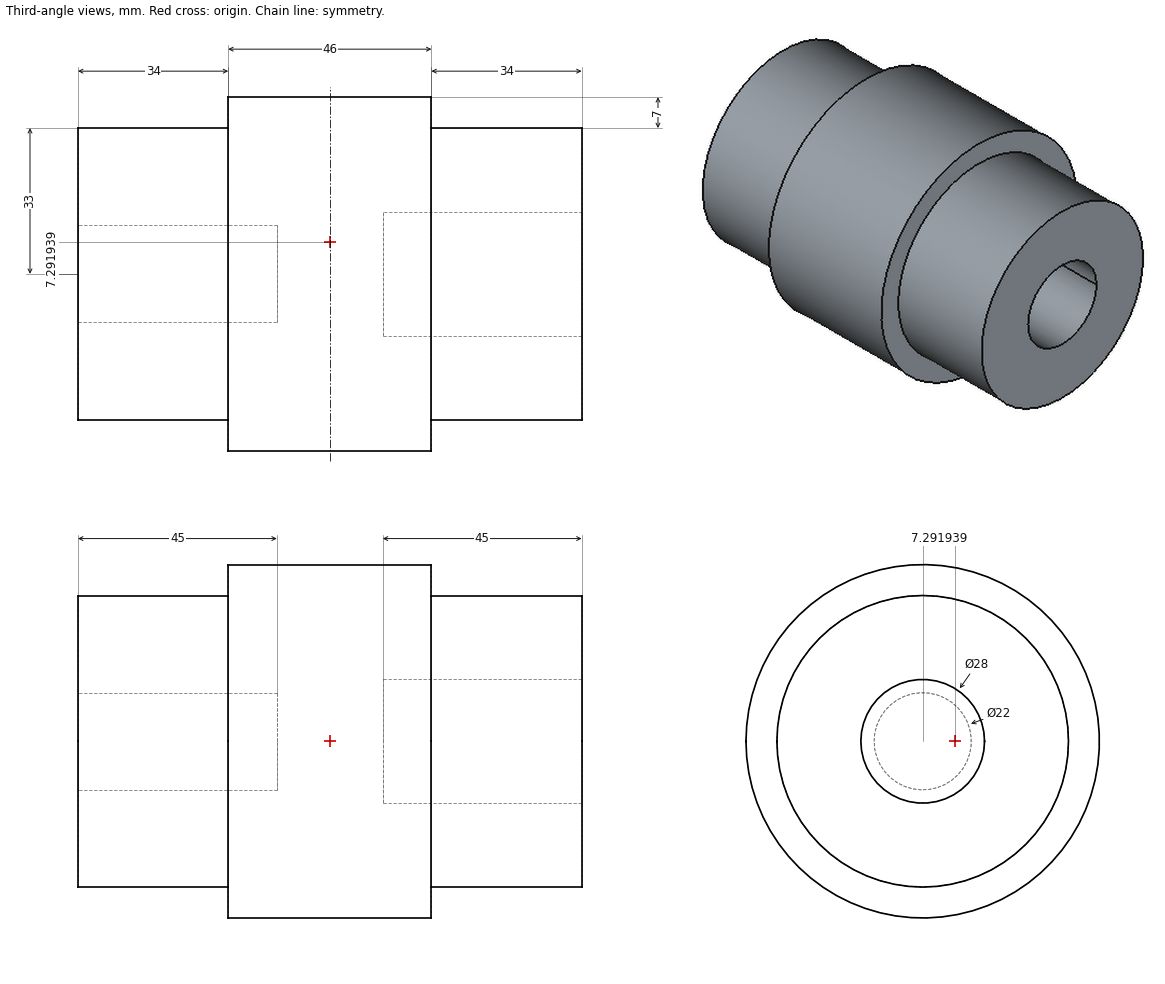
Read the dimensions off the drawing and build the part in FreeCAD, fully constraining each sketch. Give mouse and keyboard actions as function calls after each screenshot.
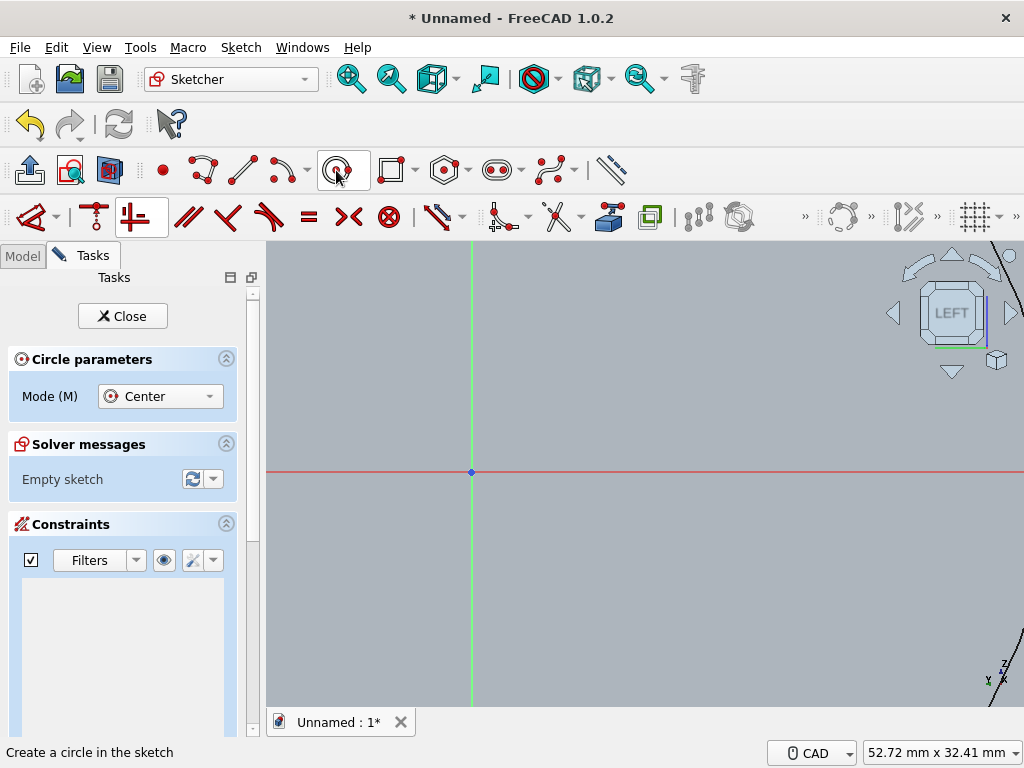
click(577, 472)
move(688, 360)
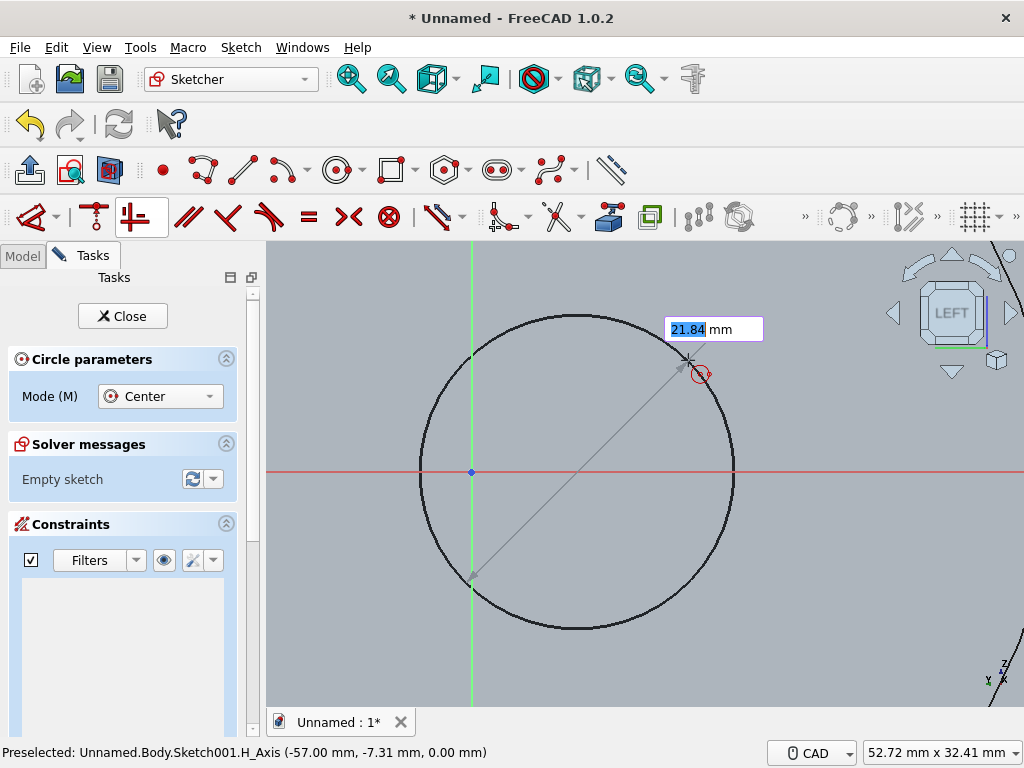
text(22)
key(Return)
key(Escape)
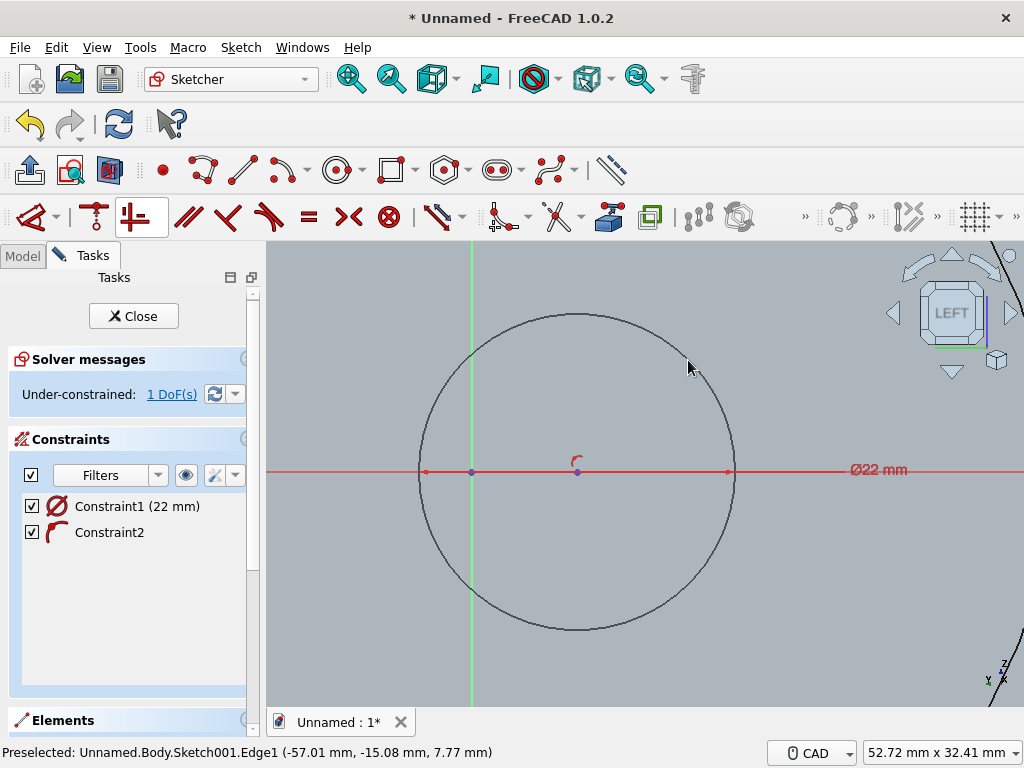
click(32, 218)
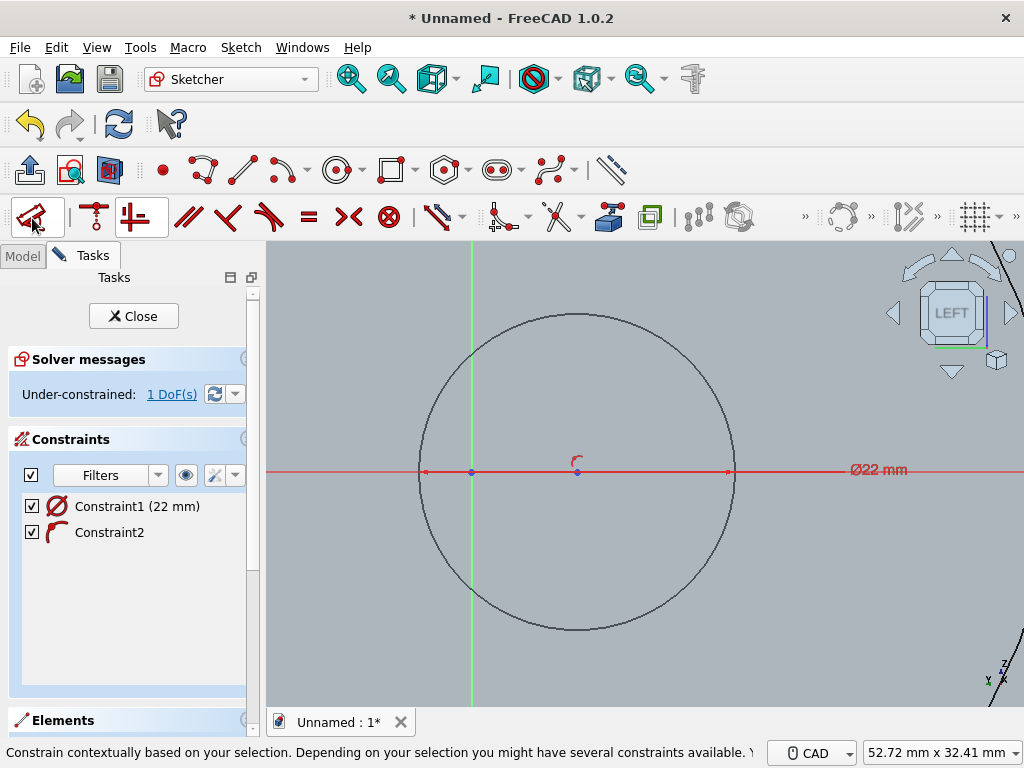
click(577, 472)
click(524, 506)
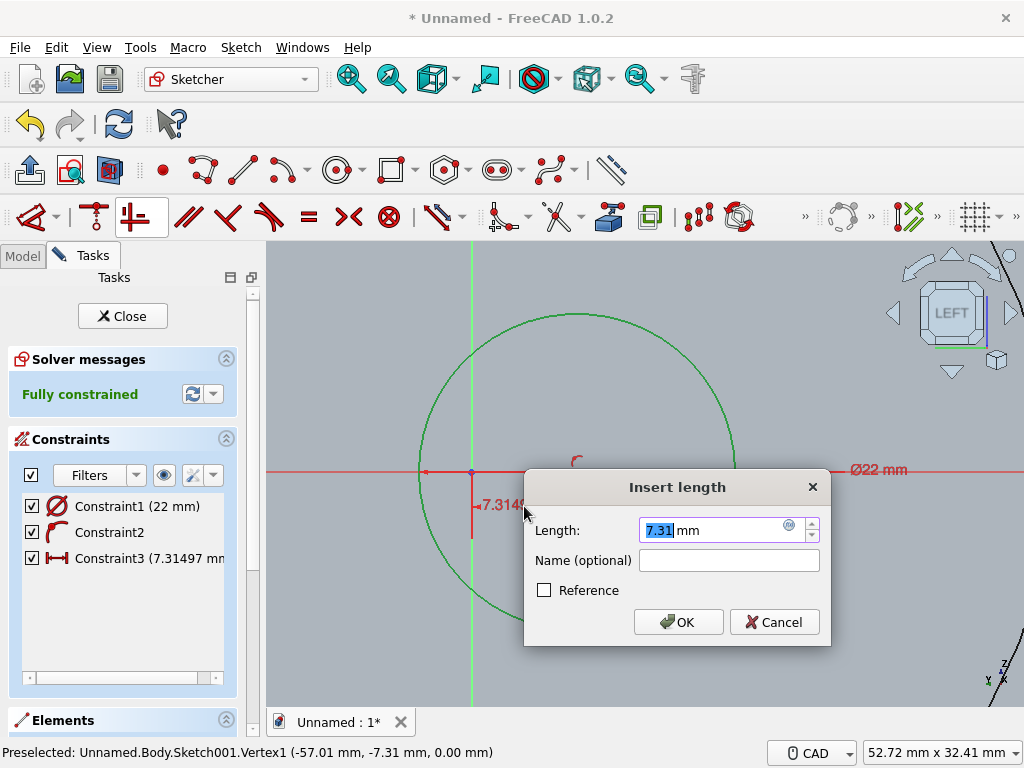
text(7.291939)
key(Return)
key(Escape)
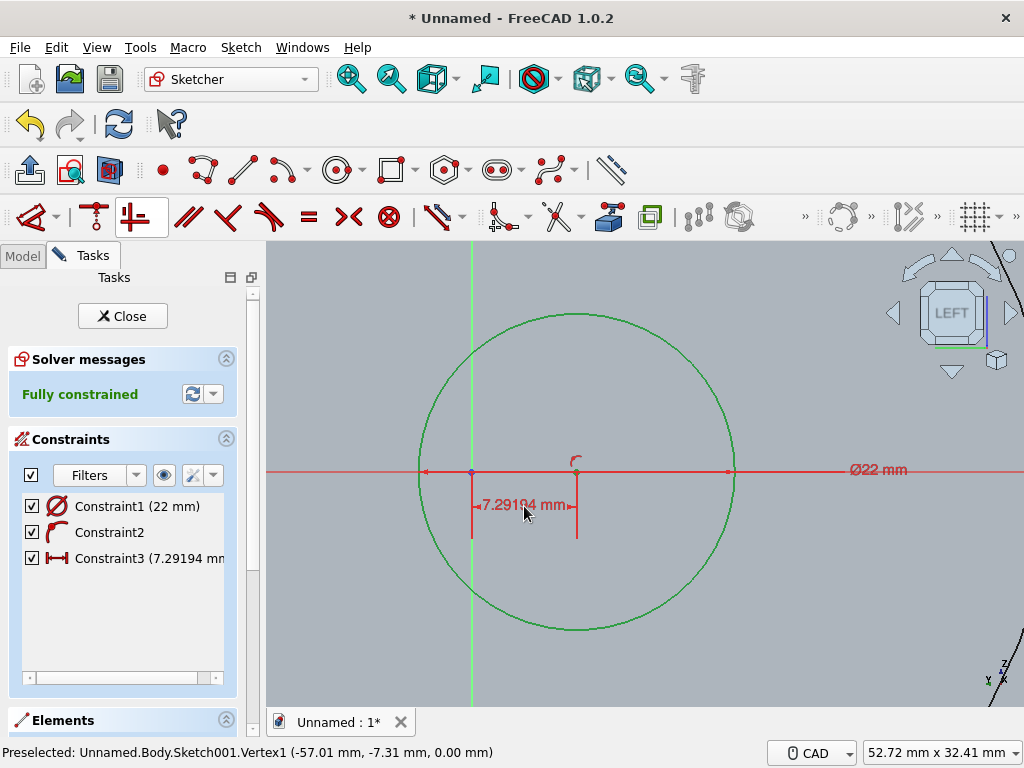
click(123, 316)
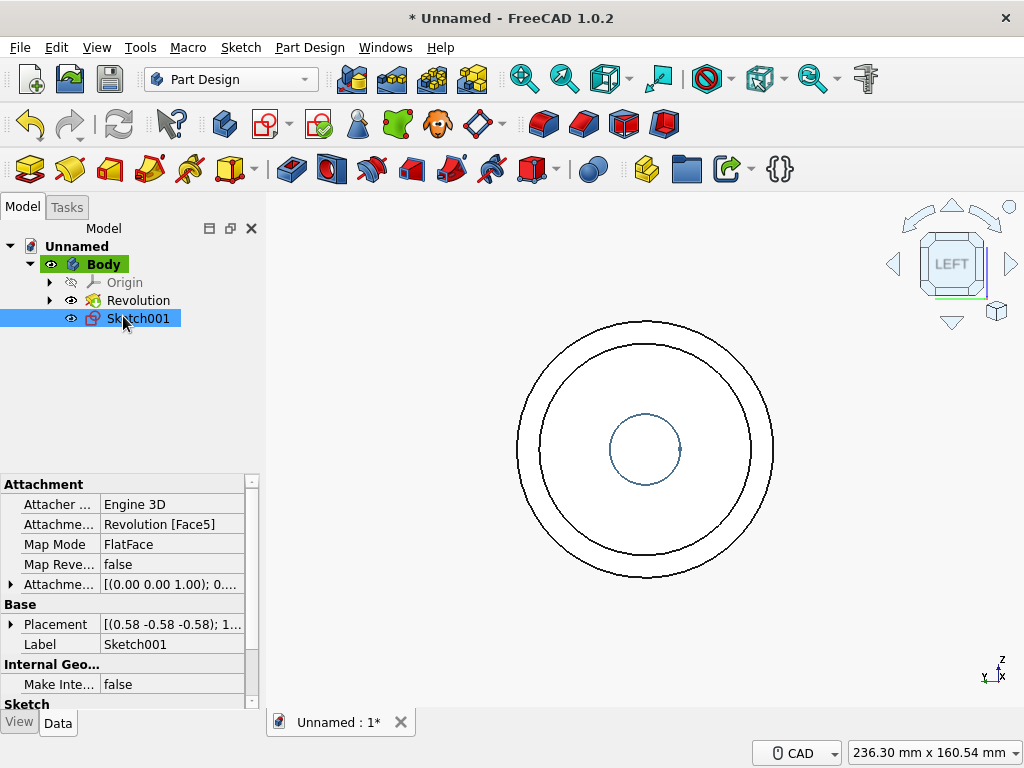
click(292, 170)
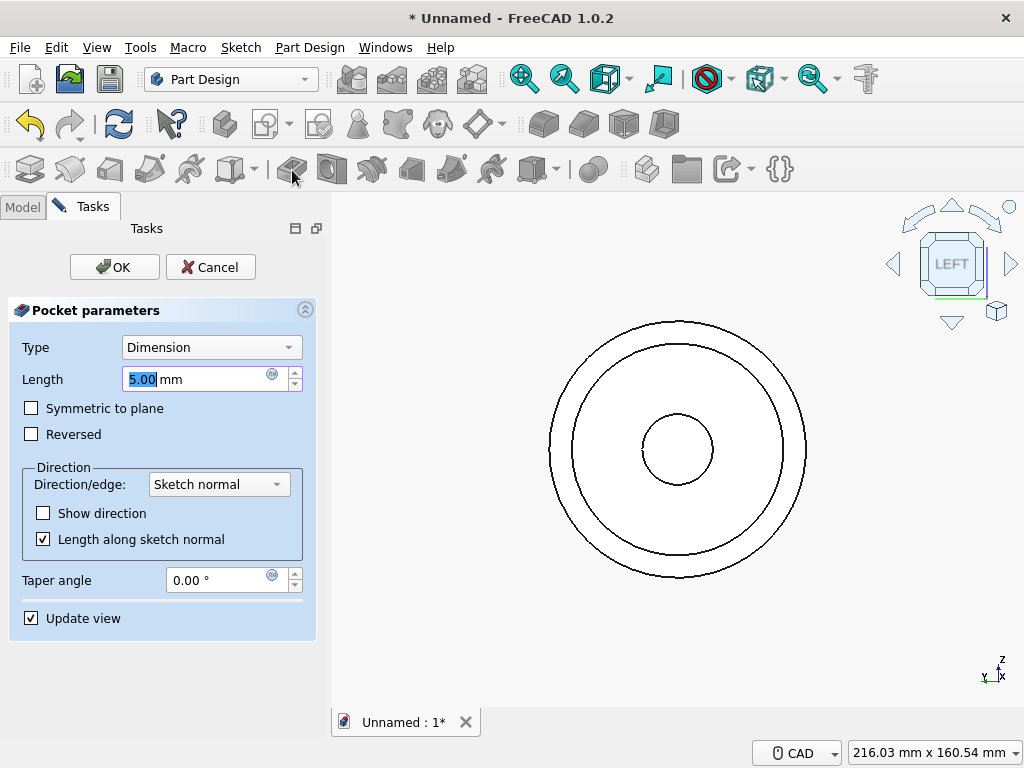
text(45)
key(Tab)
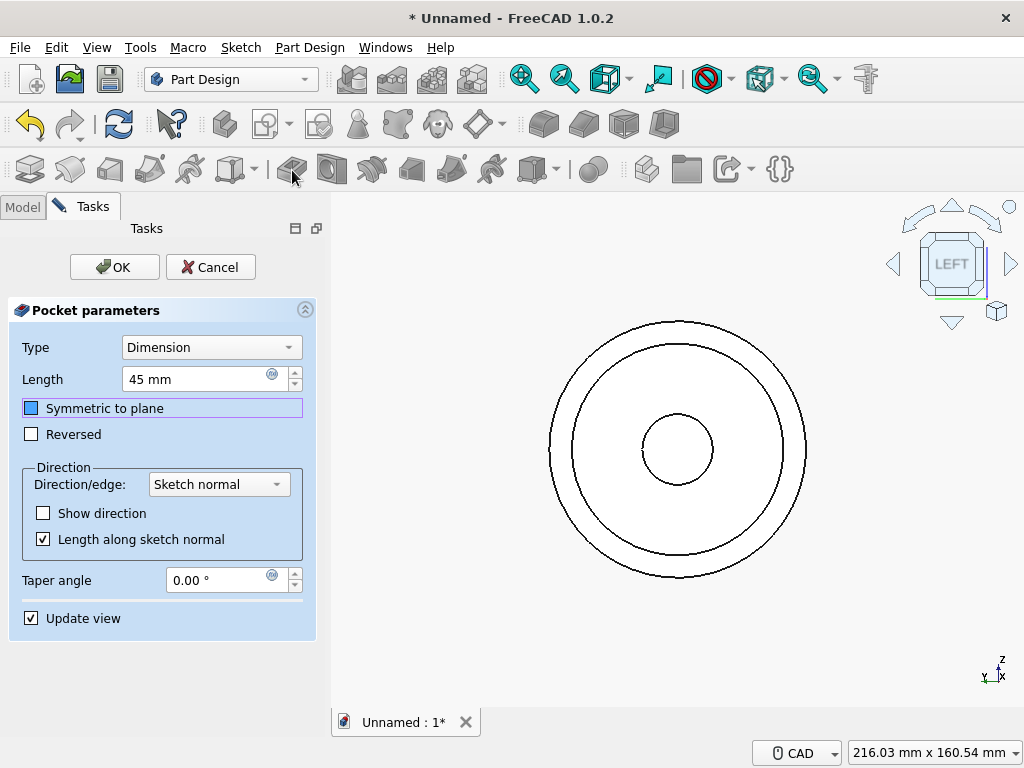
click(115, 267)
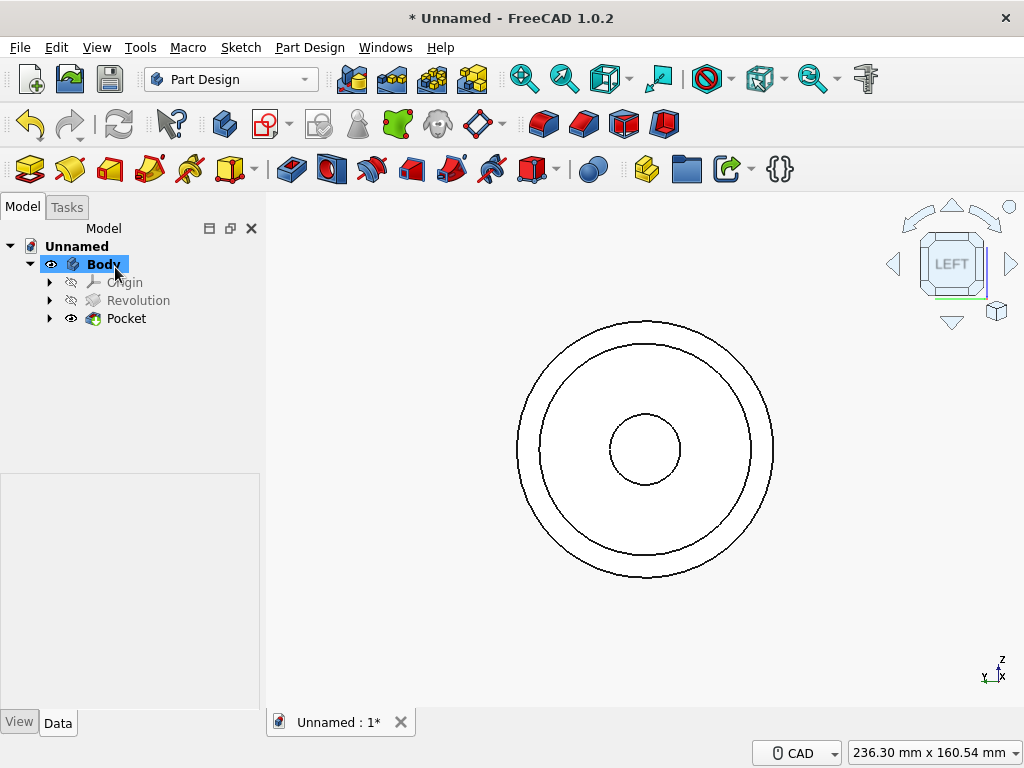
key(0)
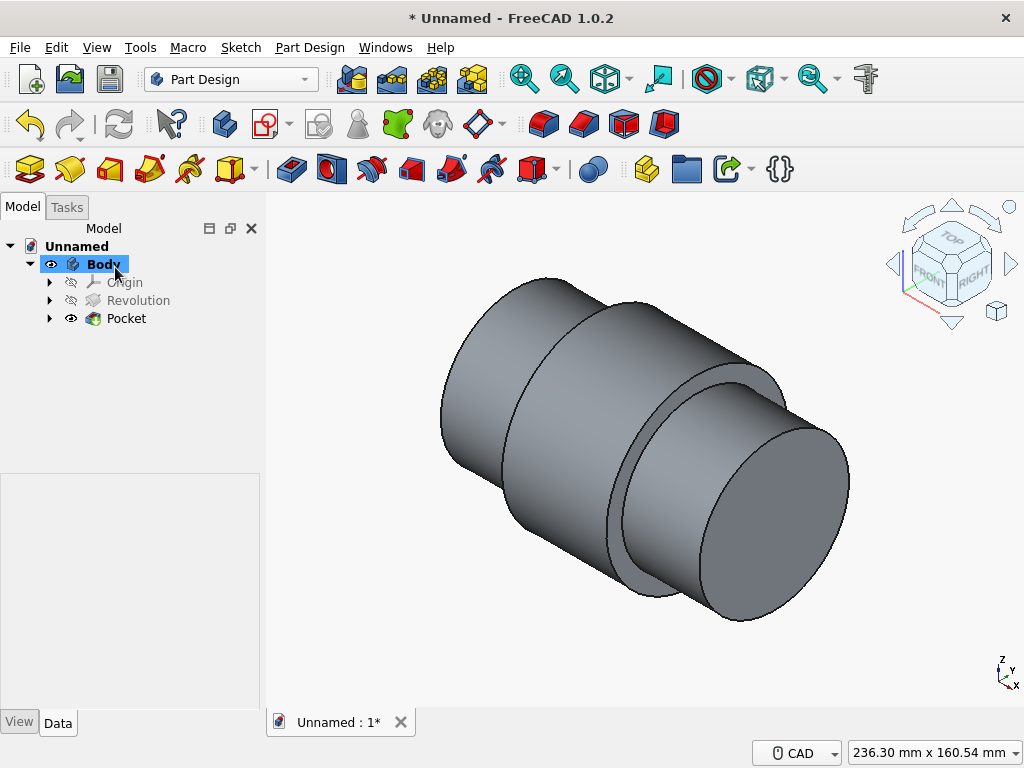
click(774, 523)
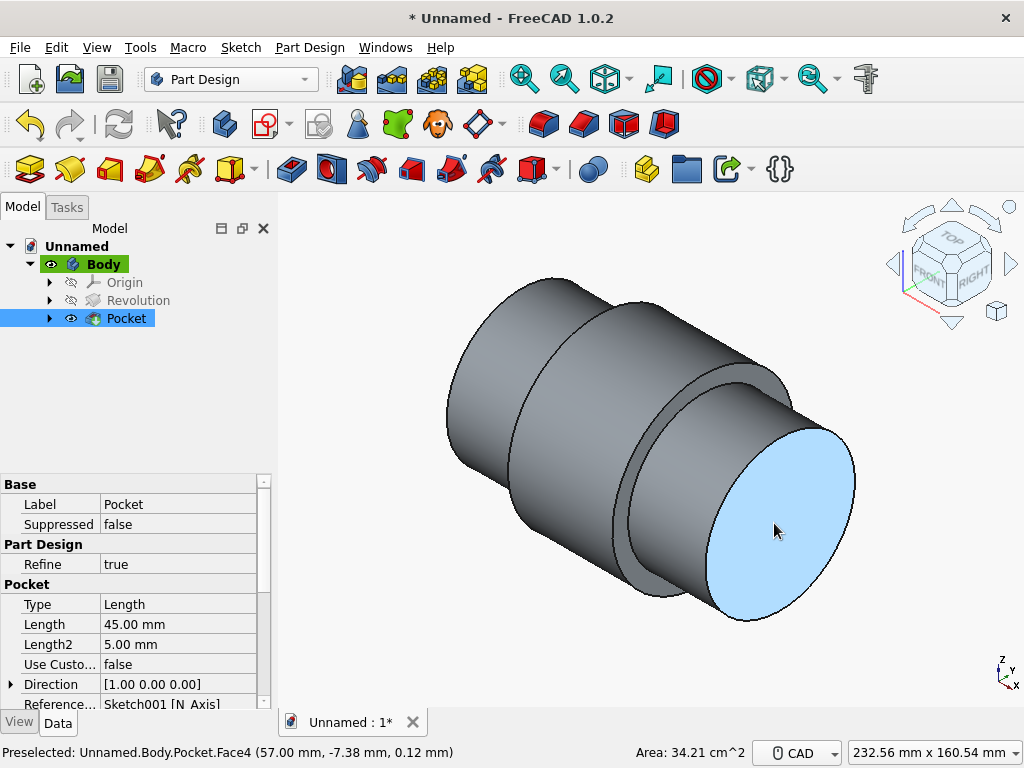
click(266, 124)